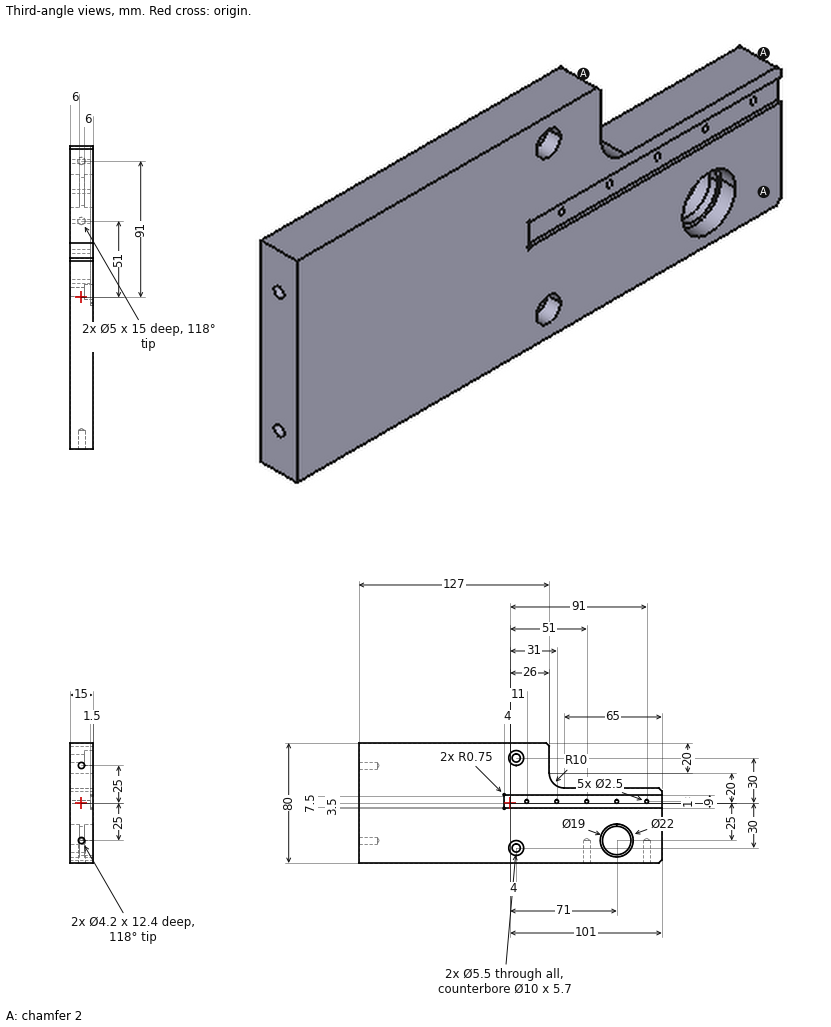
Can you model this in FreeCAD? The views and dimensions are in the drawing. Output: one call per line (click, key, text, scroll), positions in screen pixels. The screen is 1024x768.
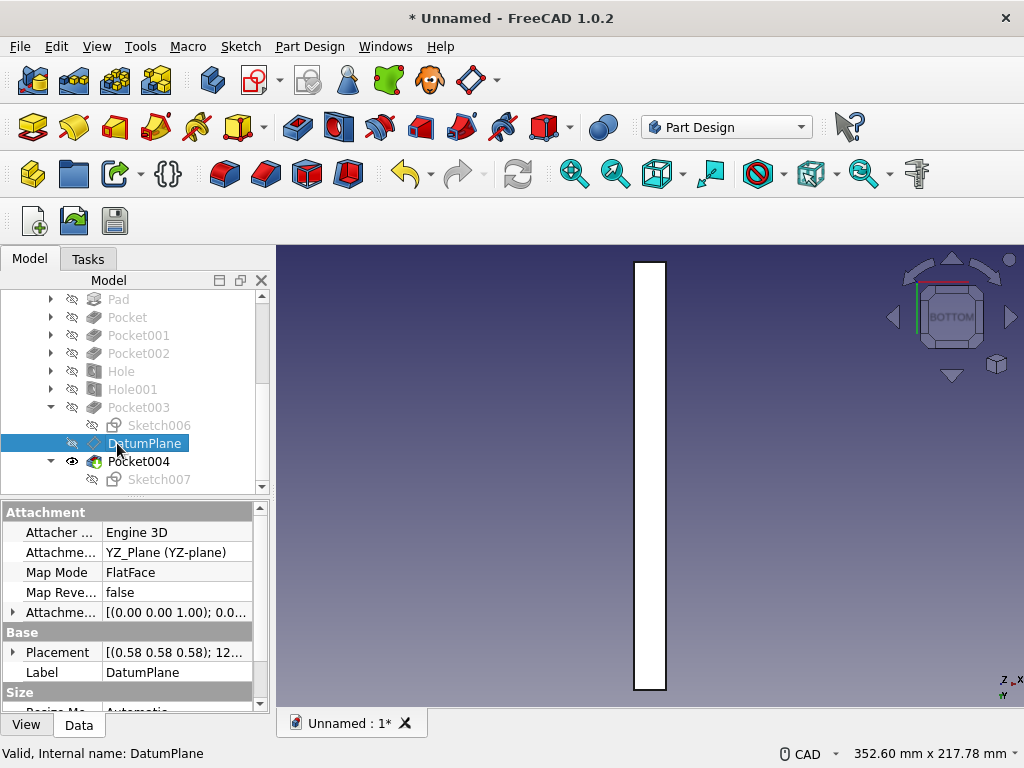
click(650, 659)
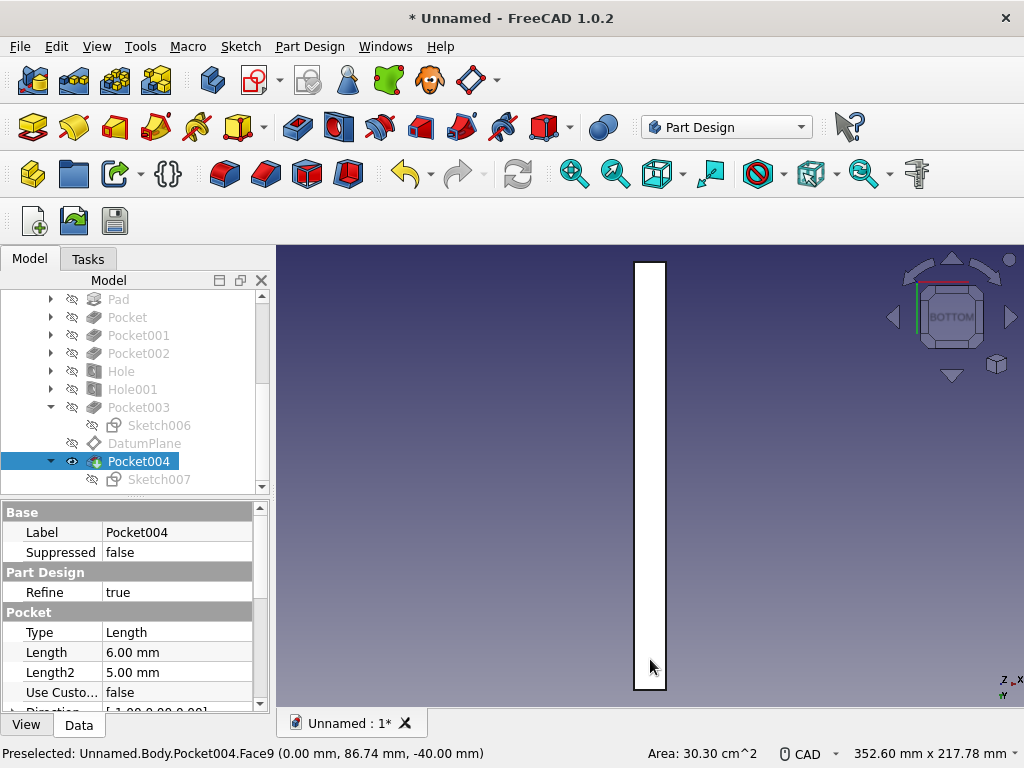
click(254, 80)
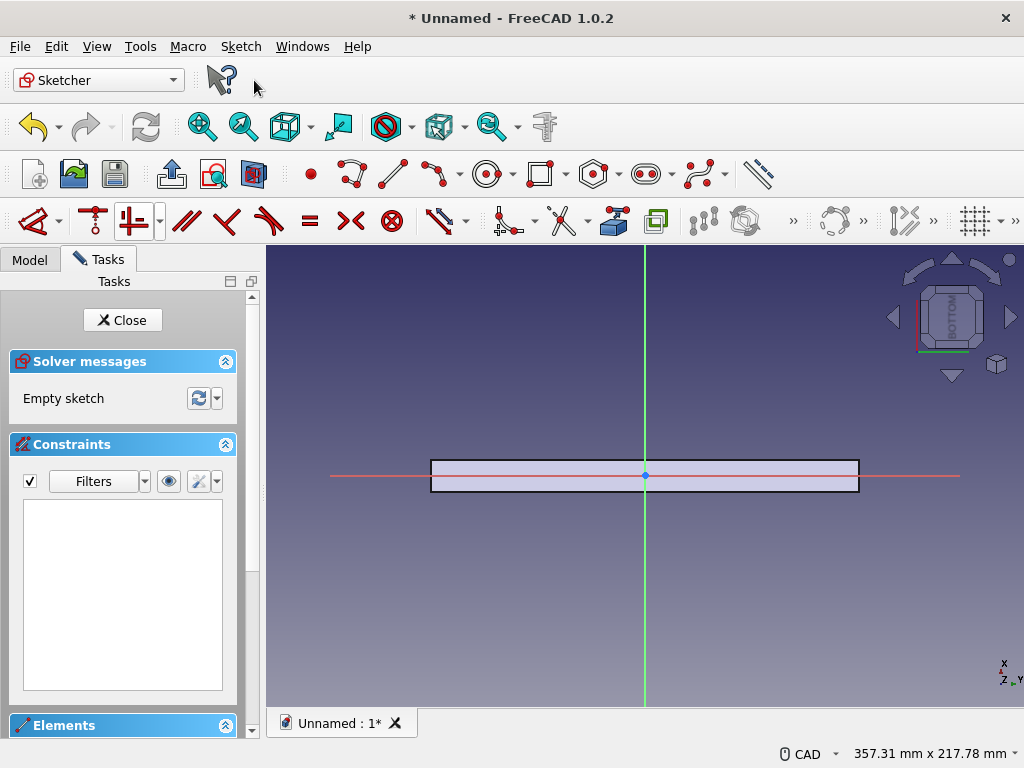
scroll(859, 476, up, 3)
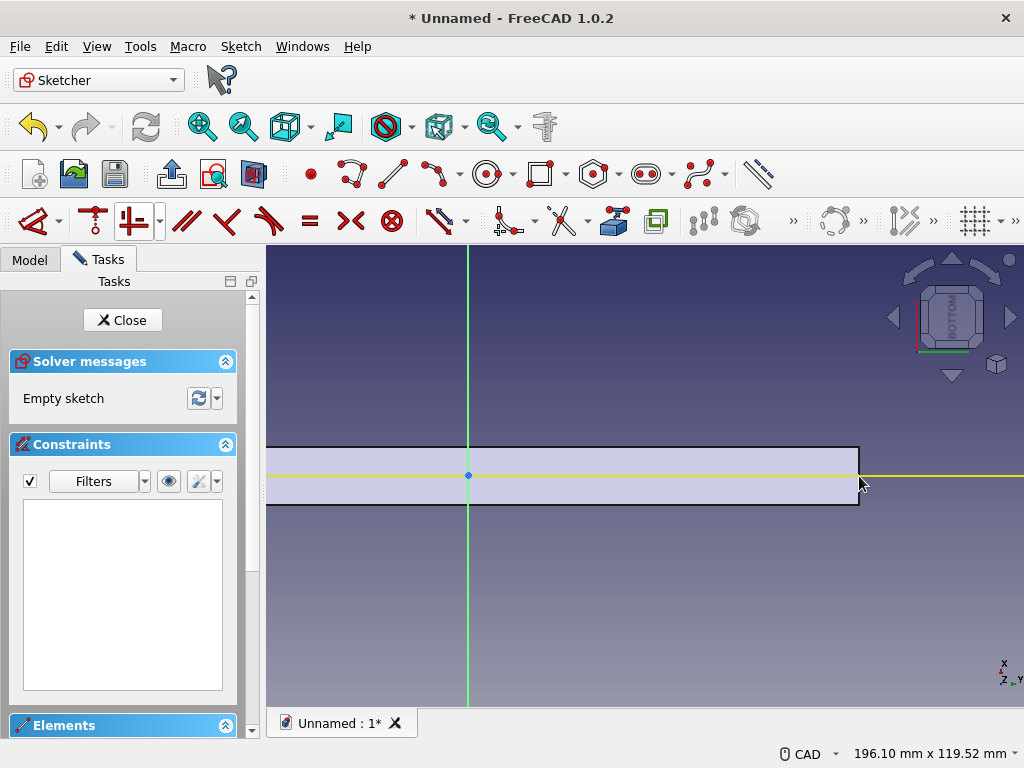
key(g)
key(c)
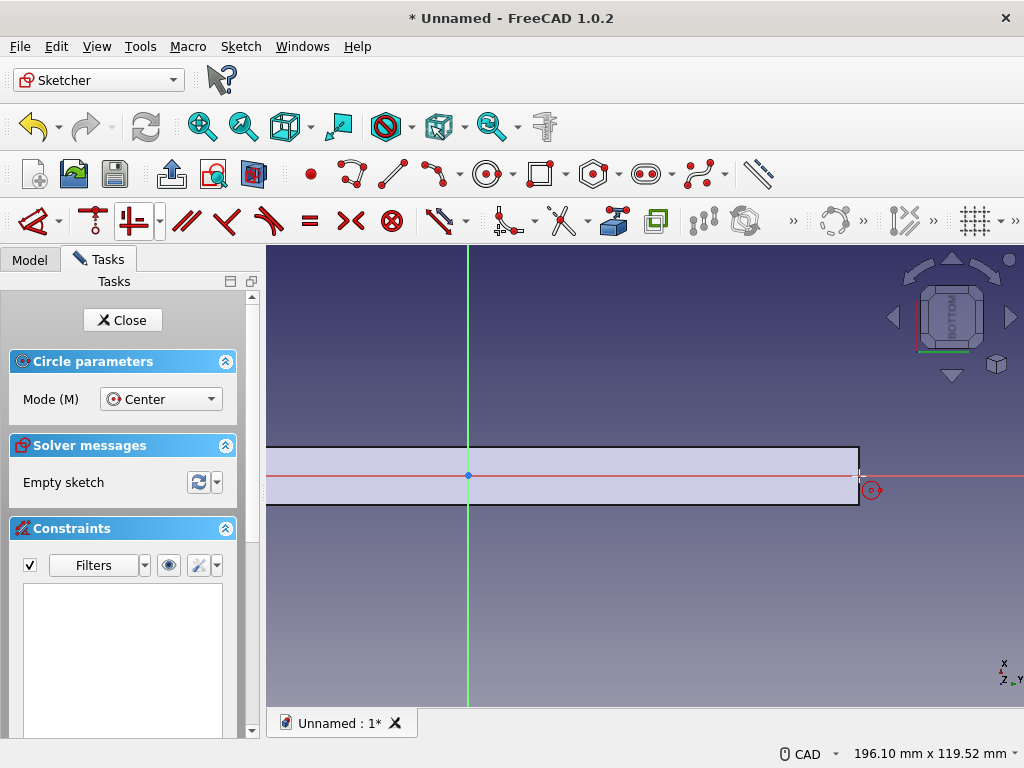
scroll(666, 476, up, 5)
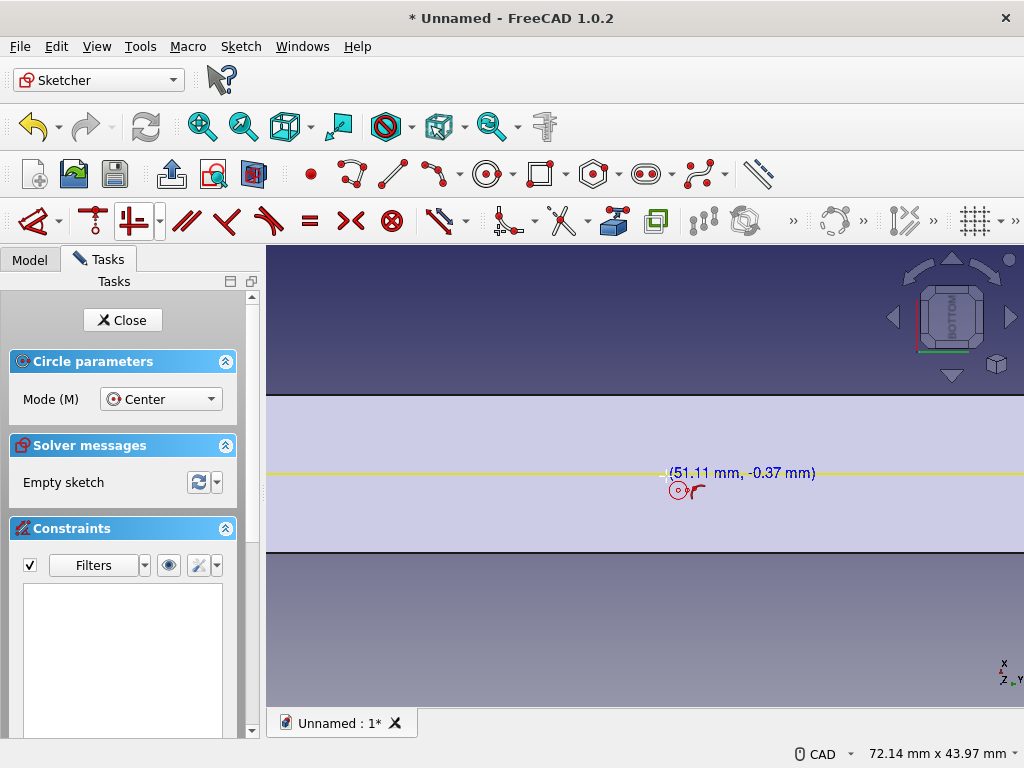
click(664, 474)
click(682, 455)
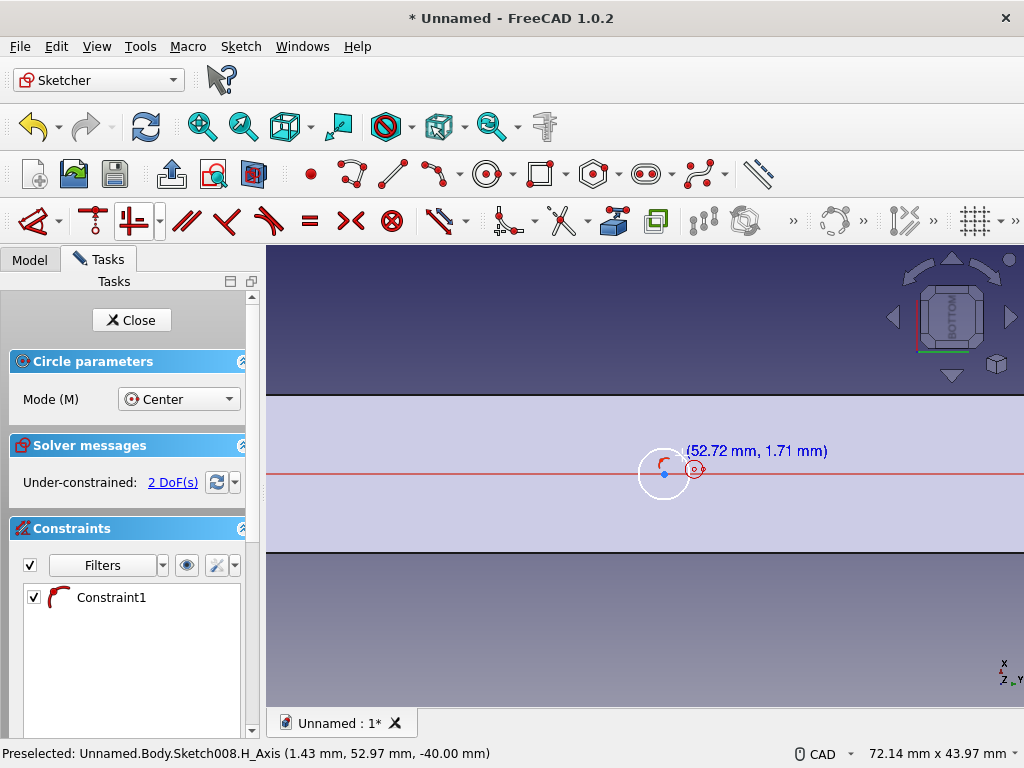
scroll(552, 477, down, 5)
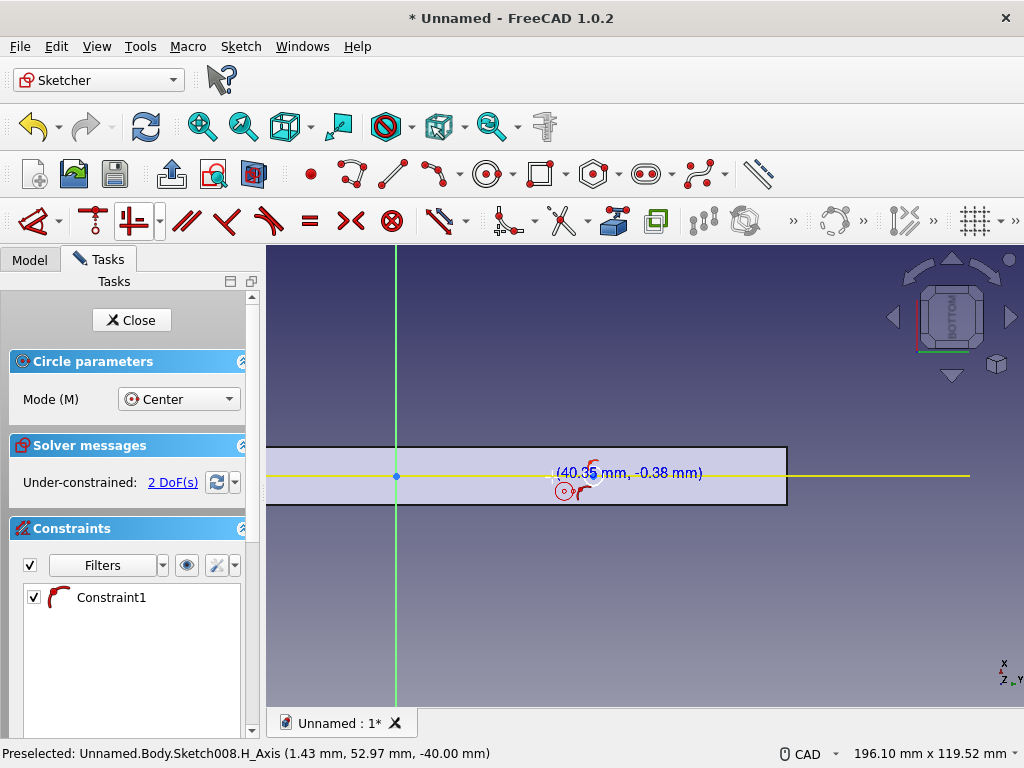
scroll(748, 476, up, 5)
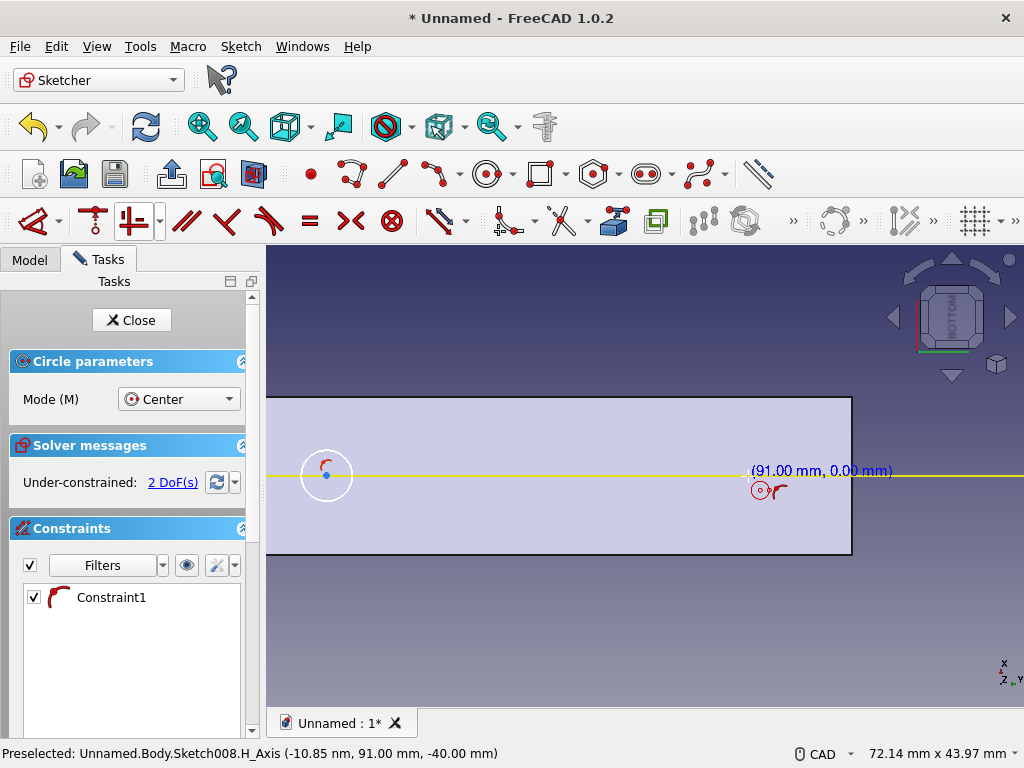
click(747, 476)
click(766, 457)
key(Escape)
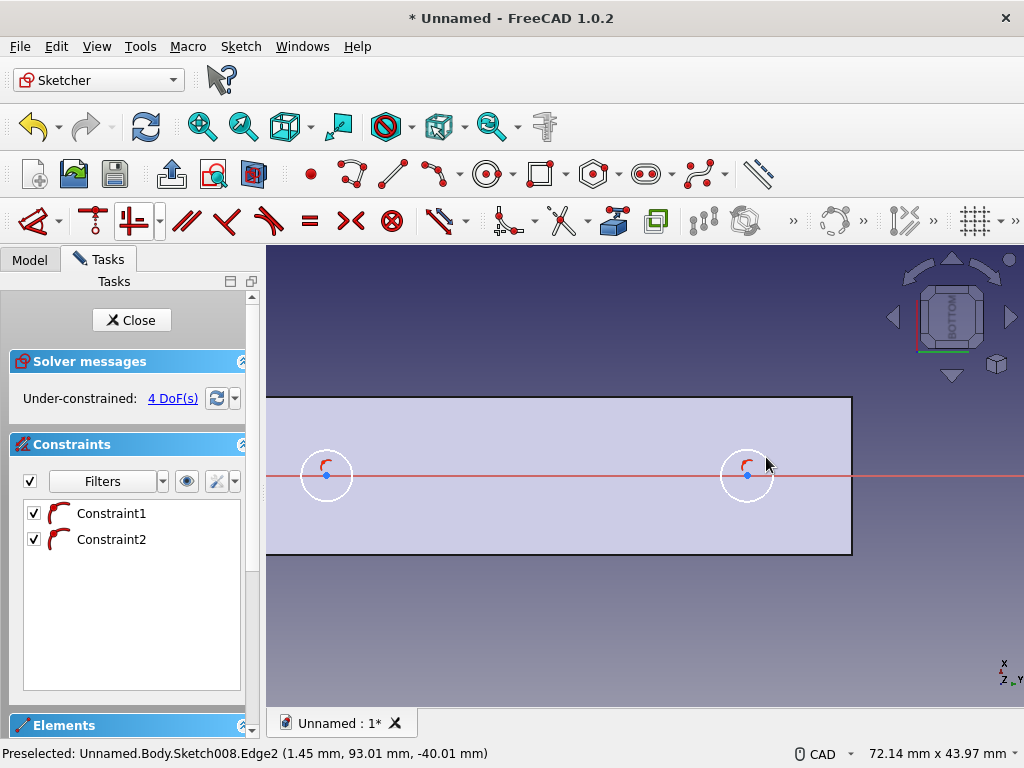
click(345, 458)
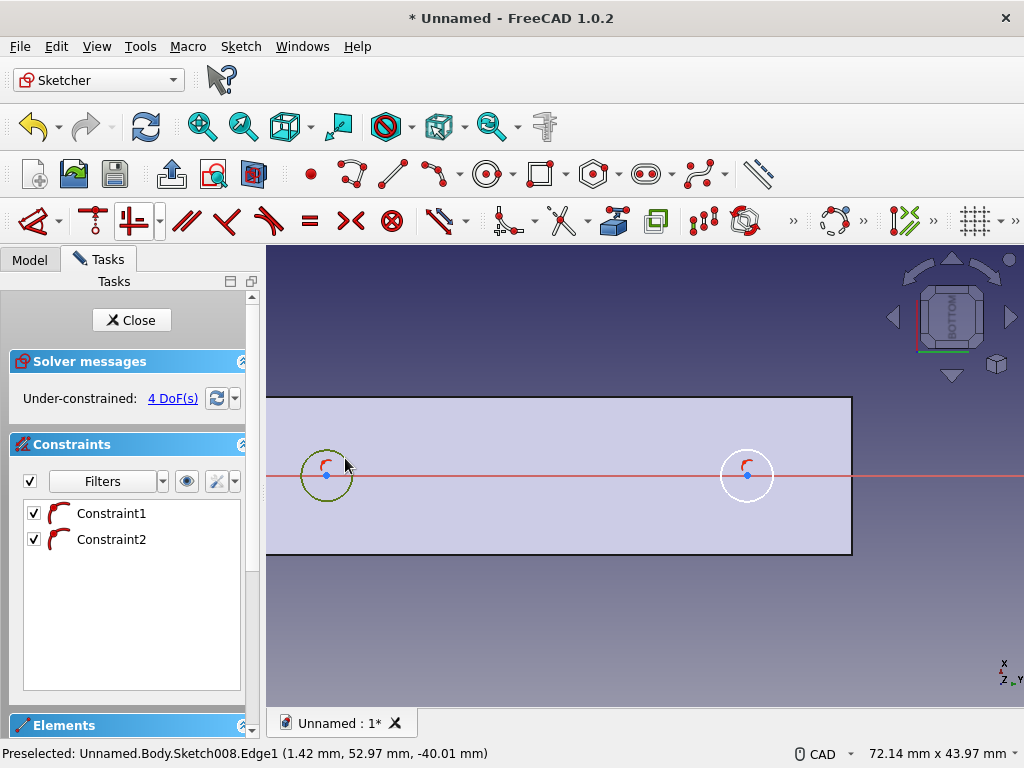
click(765, 457)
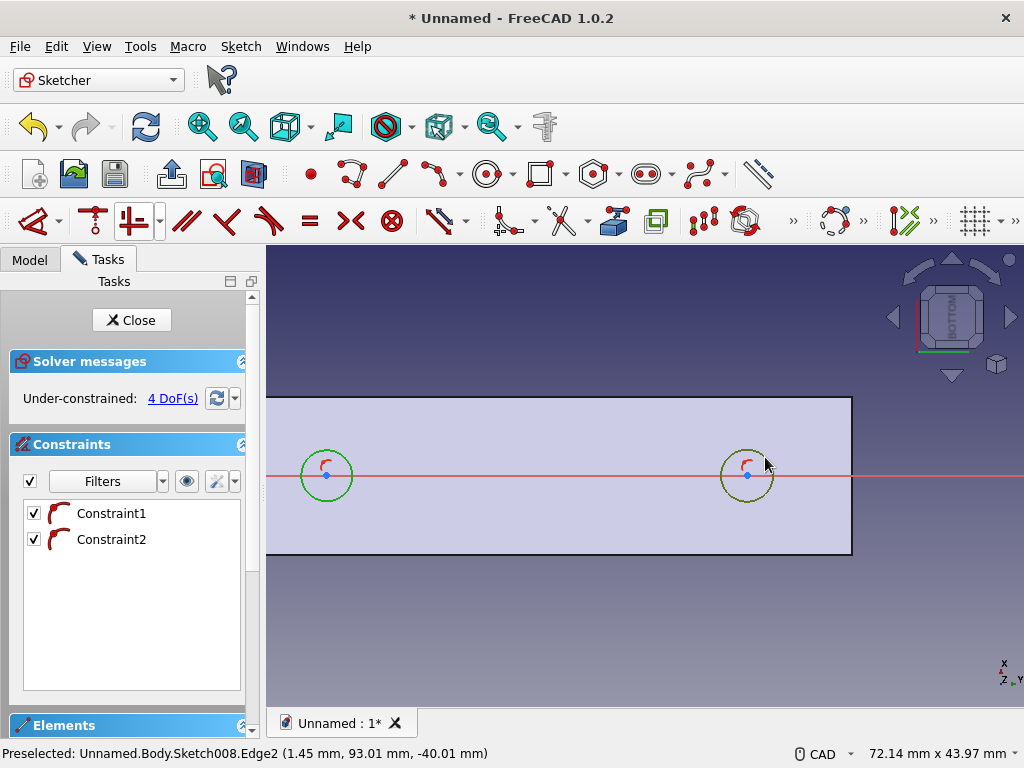
click(310, 222)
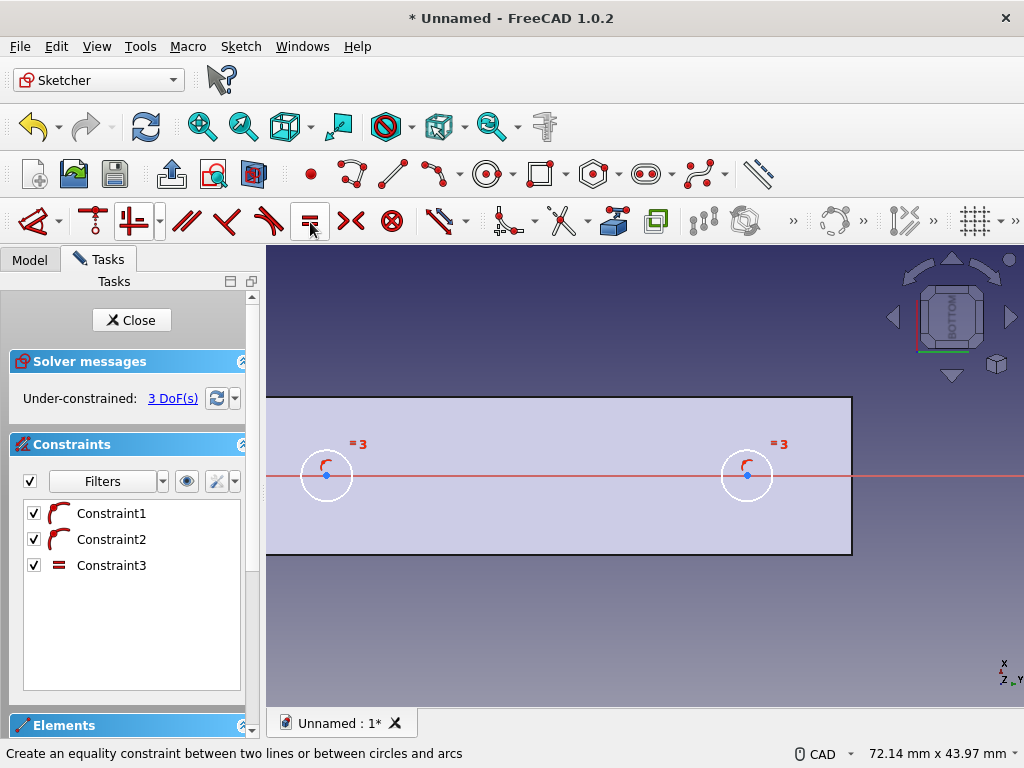
click(32, 222)